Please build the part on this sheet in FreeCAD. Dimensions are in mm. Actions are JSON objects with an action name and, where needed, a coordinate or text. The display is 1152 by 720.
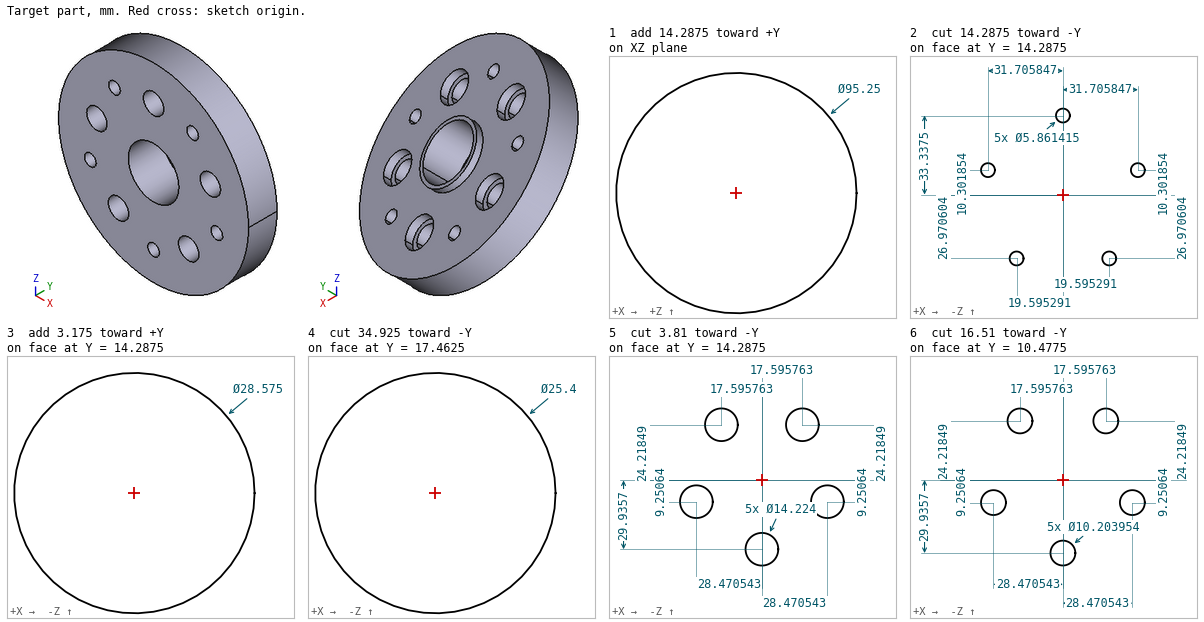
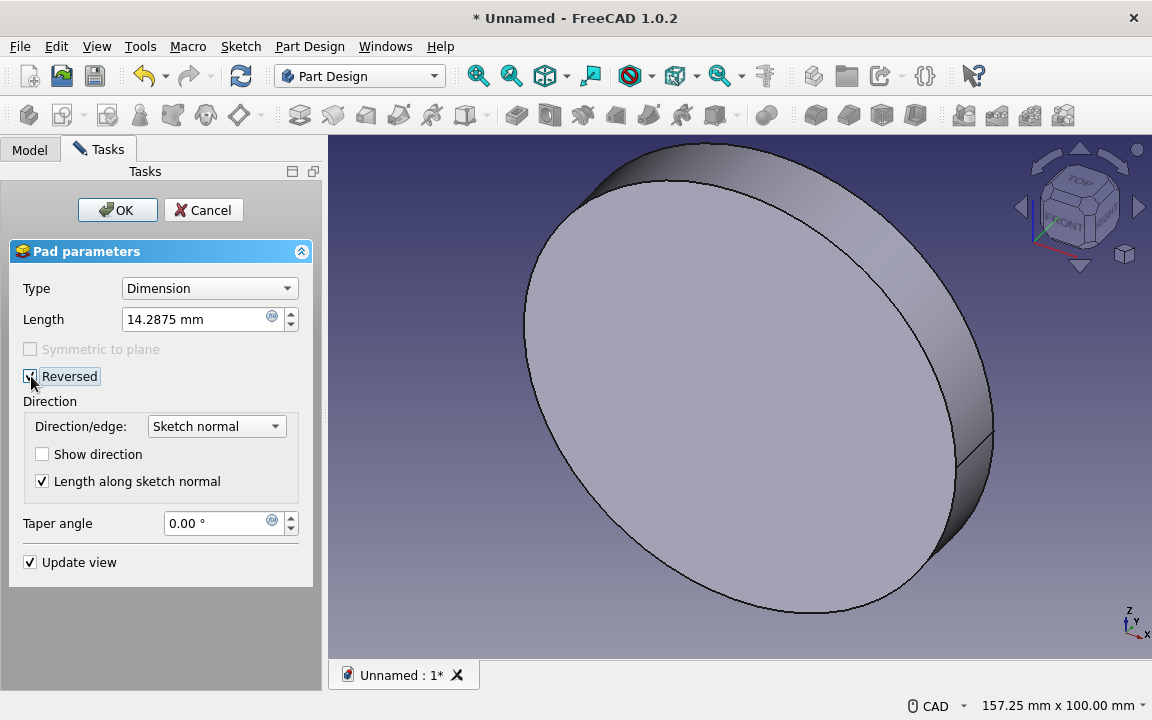
{"action": "left_click", "coordinate": [118, 210]}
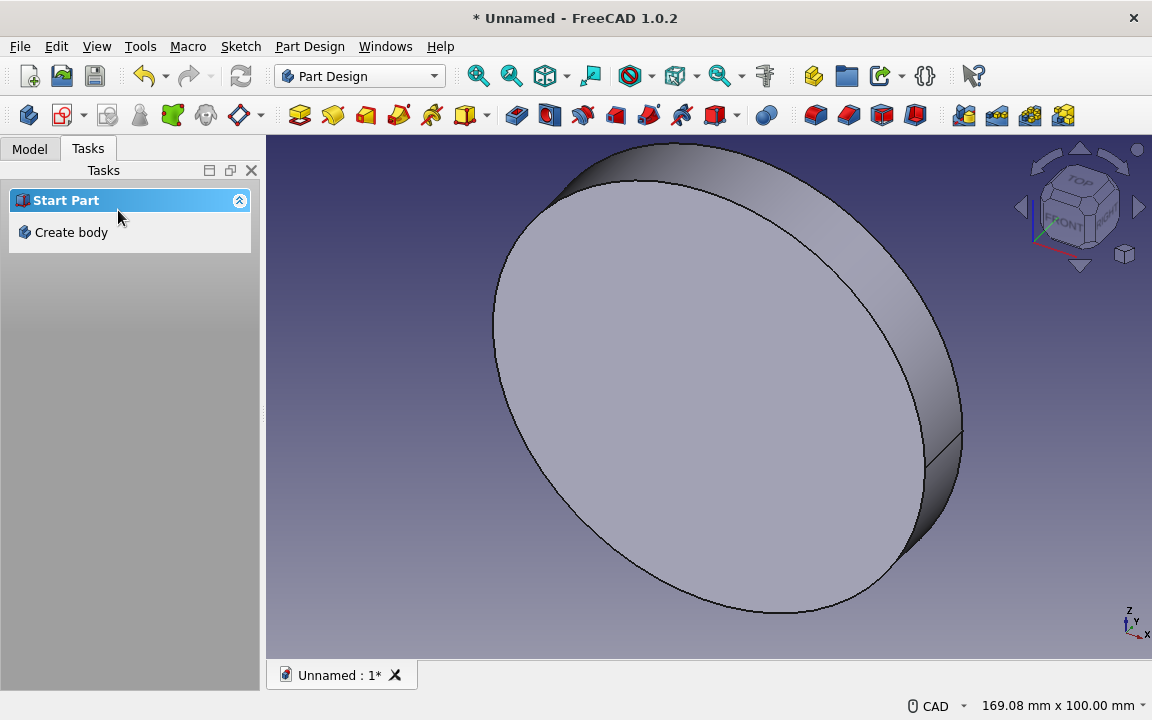
{"action": "left_click", "coordinate": [479, 76]}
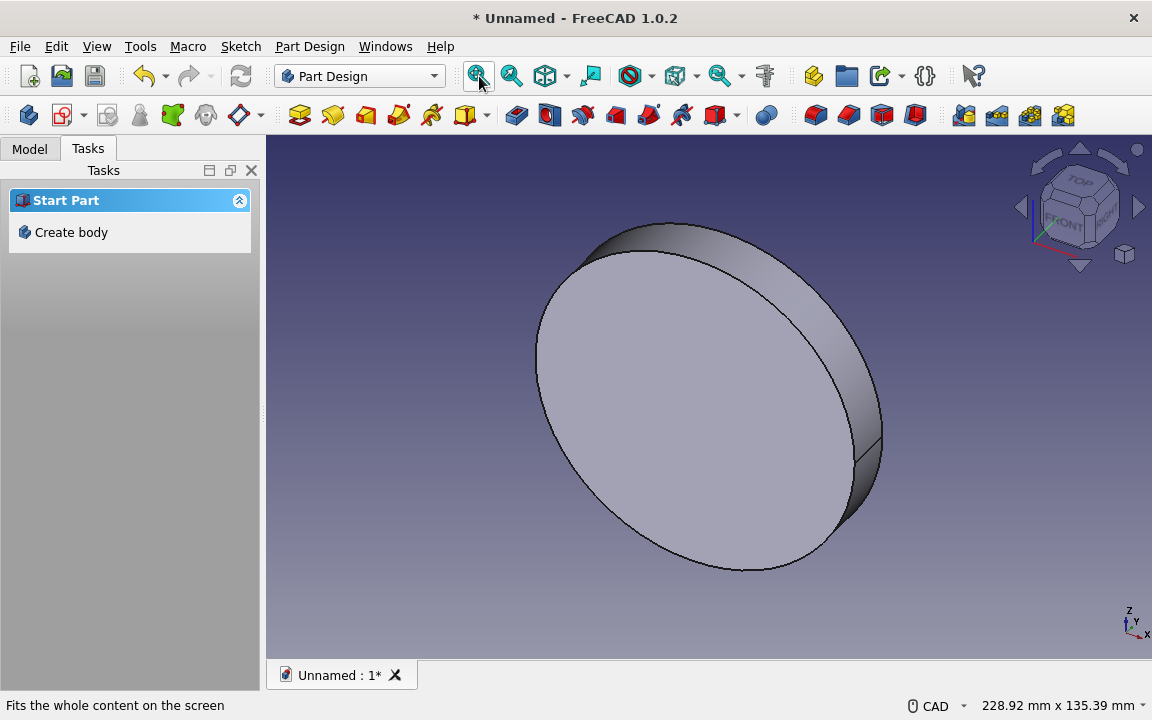
{"action": "key", "text": "4"}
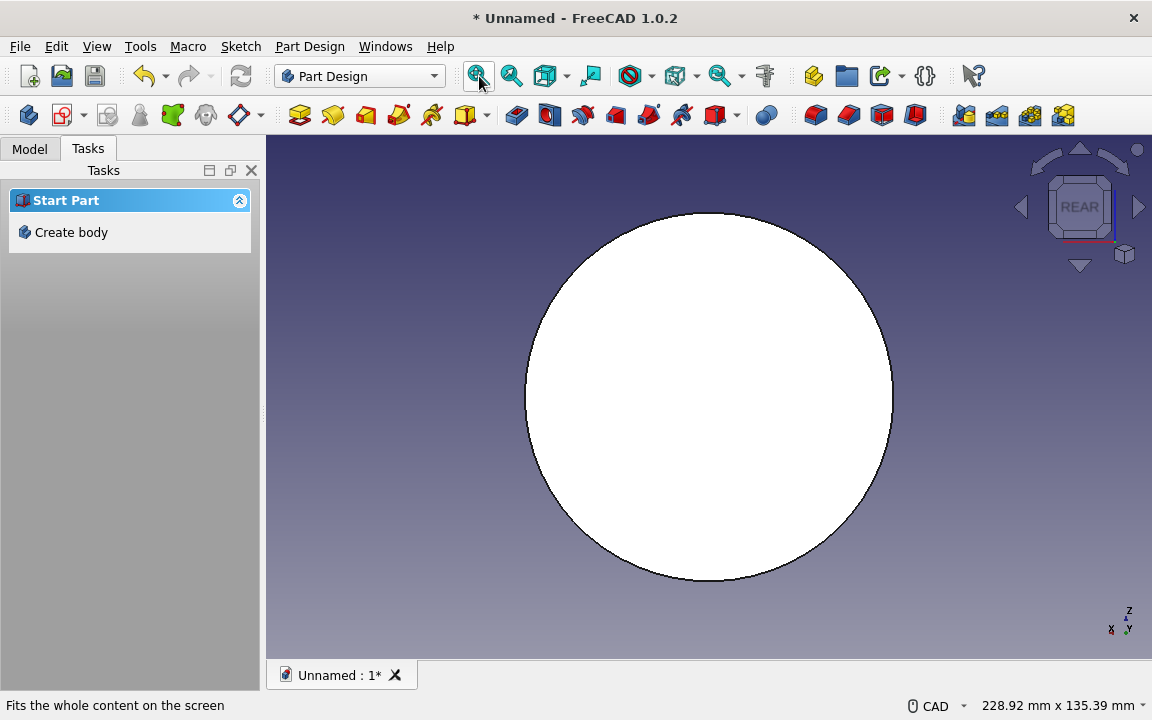
{"action": "left_click", "coordinate": [709, 396]}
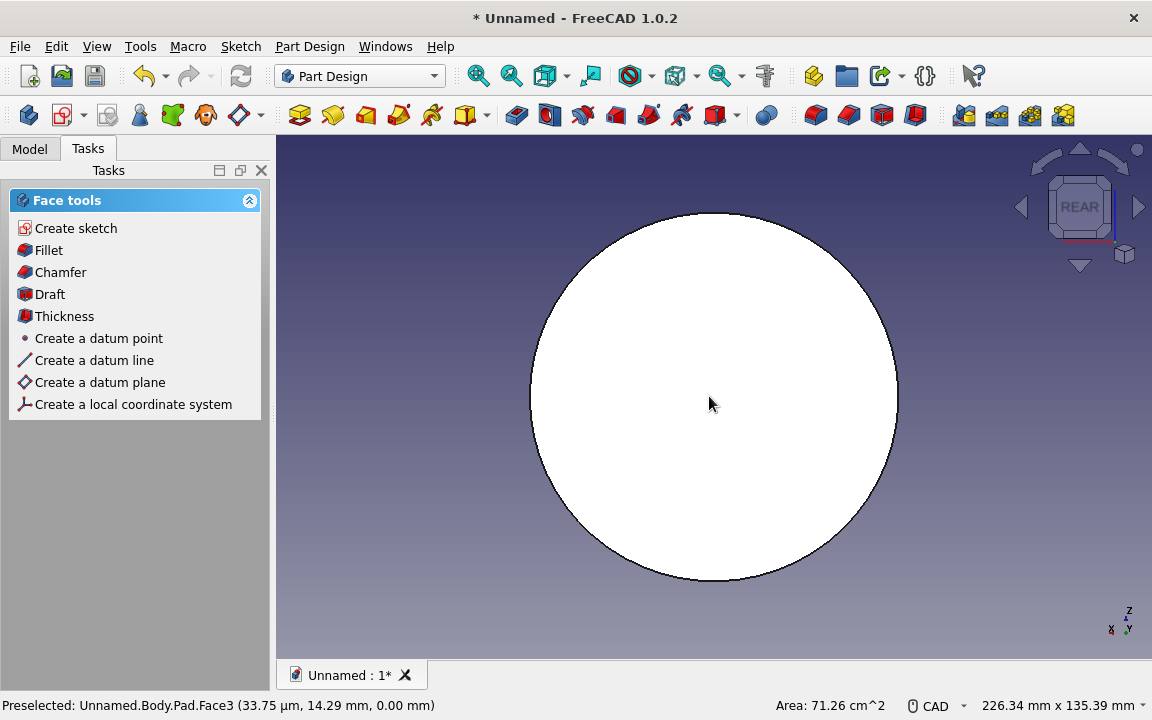
{"action": "left_click", "coordinate": [62, 116]}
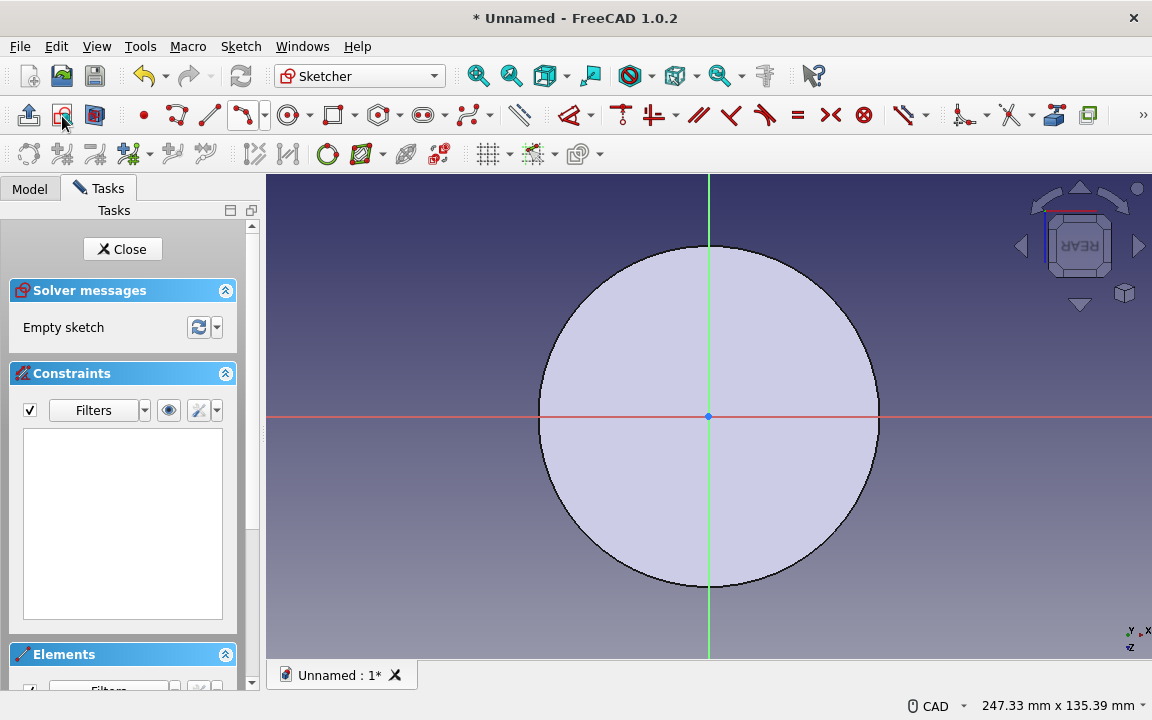
{"action": "left_click", "coordinate": [288, 116]}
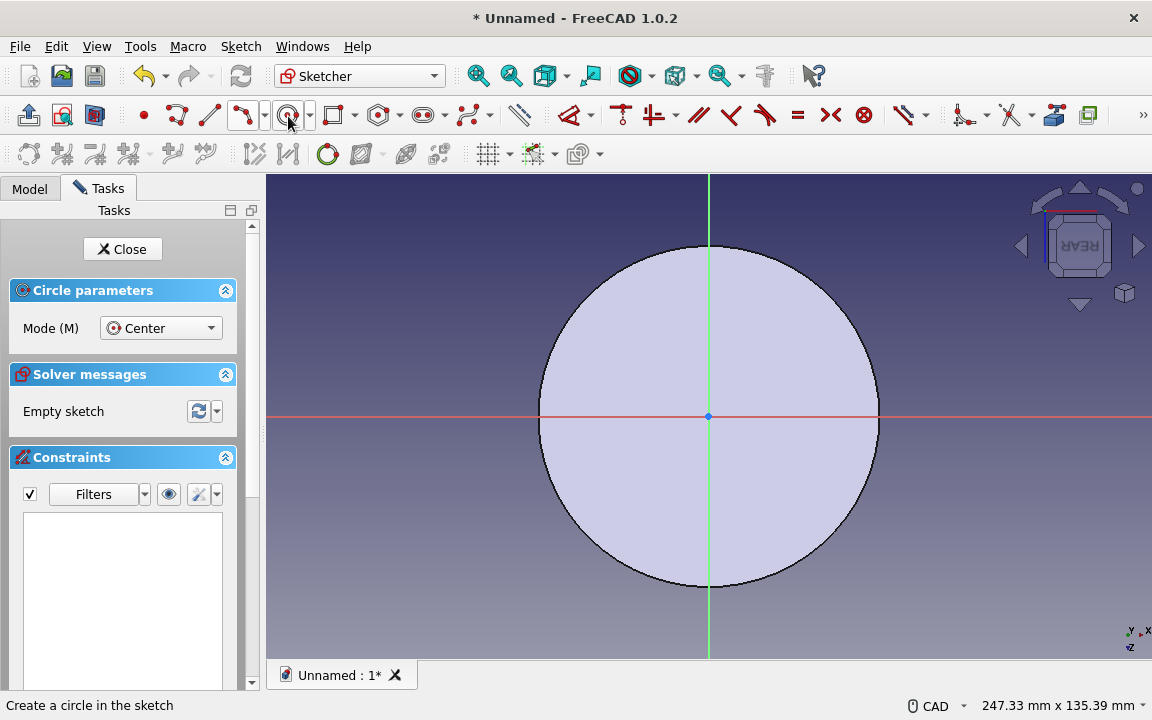
{"action": "scroll", "coordinate": [709, 297], "scroll_direction": "up", "scroll_amount": 4}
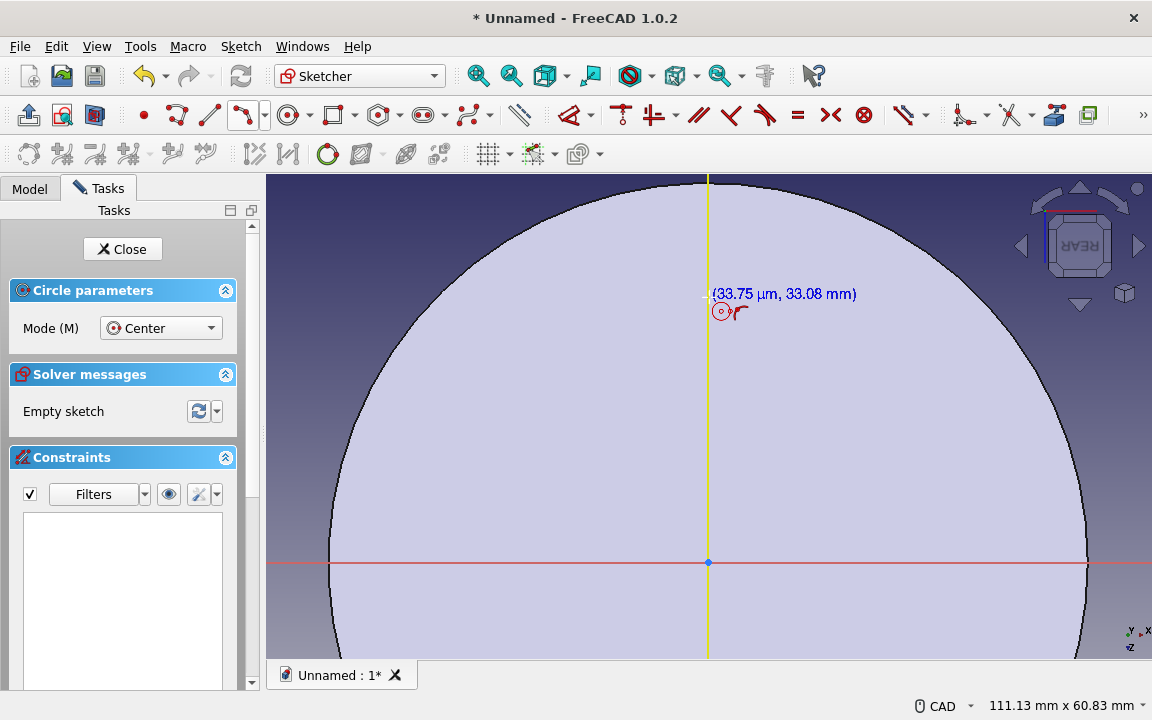
{"action": "left_click", "coordinate": [708, 297]}
{"action": "mouse_move", "coordinate": [725, 280]}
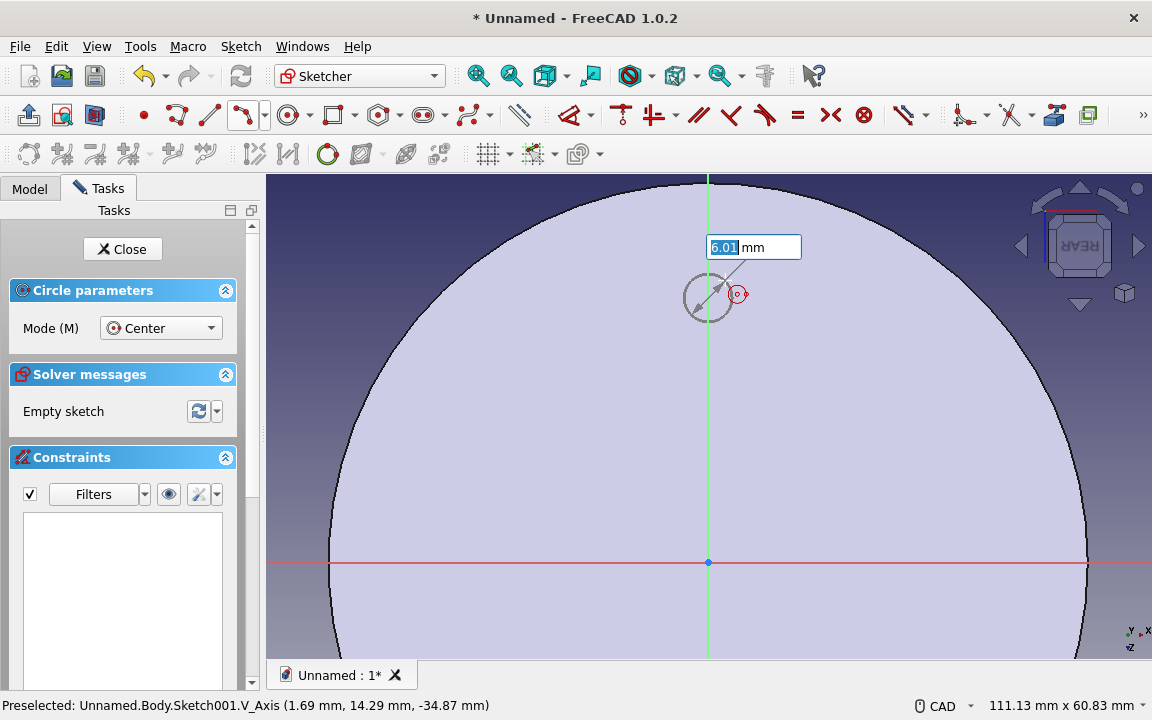
{"action": "type", "text": "5.861415"}
{"action": "key", "text": "Return"}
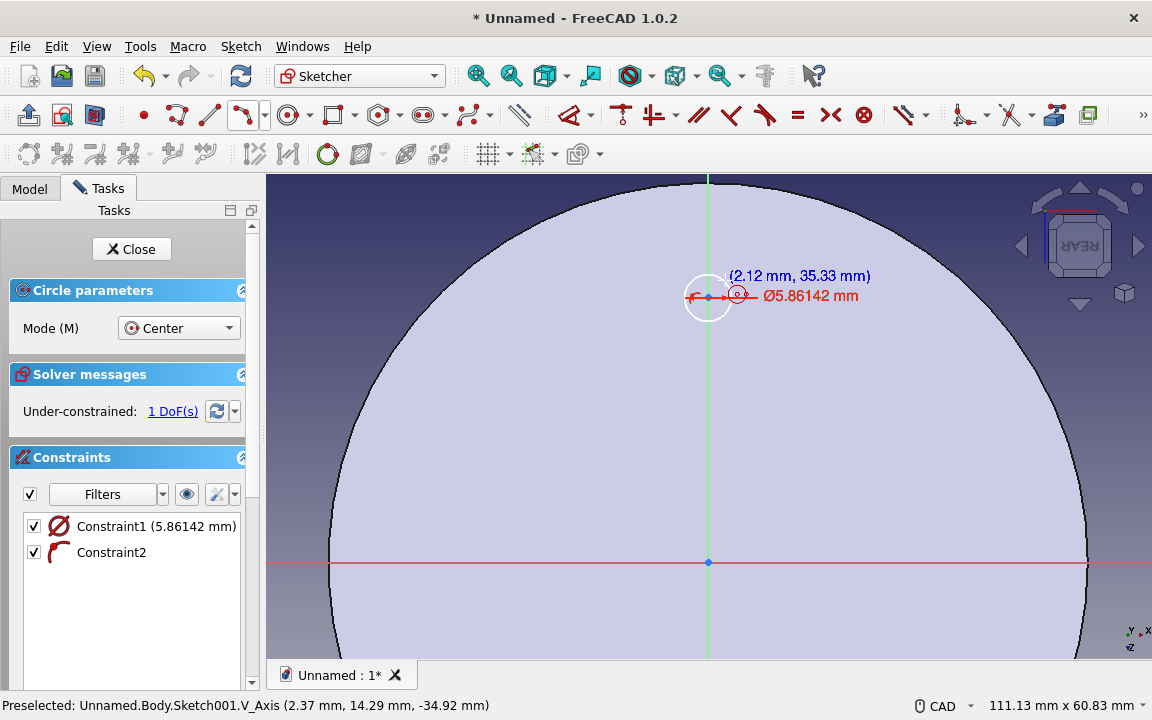
{"action": "left_click", "coordinate": [961, 481]}
{"action": "mouse_move", "coordinate": [977, 464]}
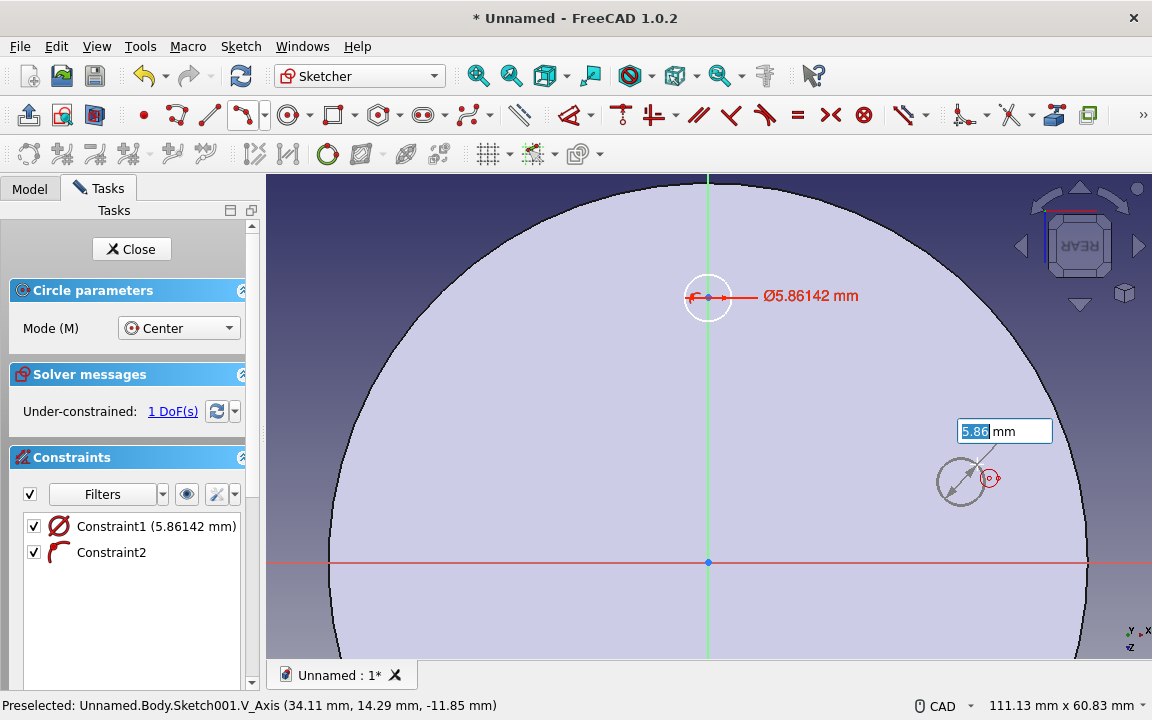
{"action": "type", "text": "5.861415"}
{"action": "key", "text": "Return"}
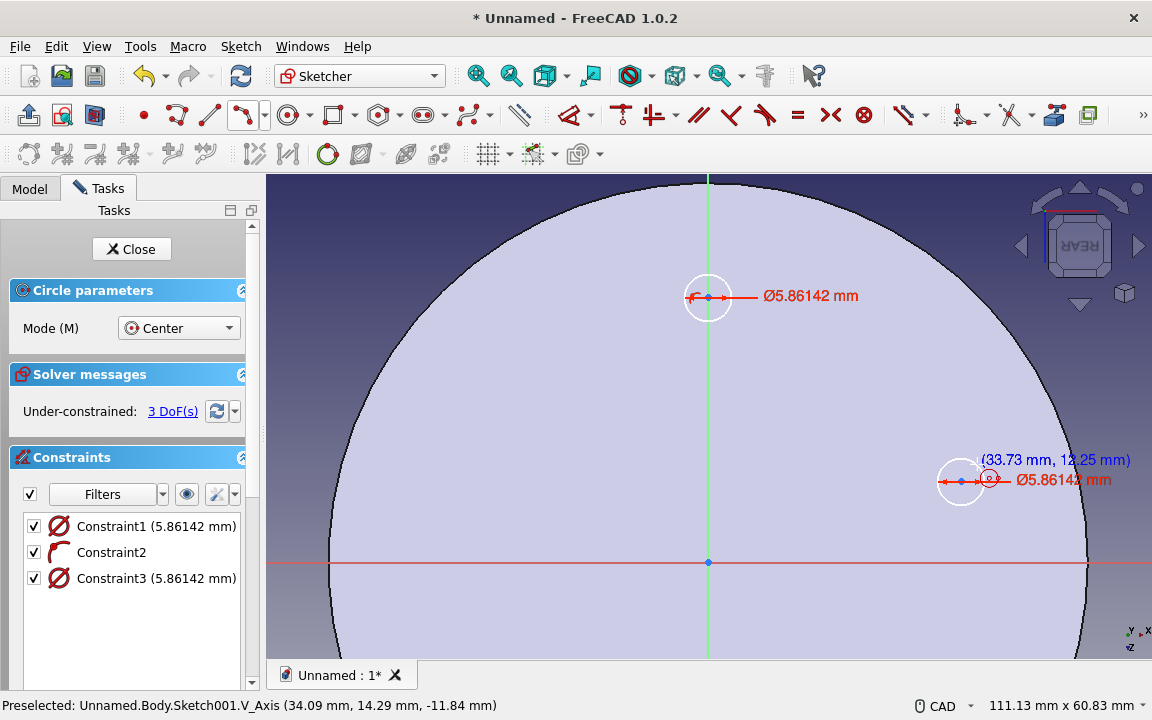
{"action": "scroll", "coordinate": [558, 270], "scroll_direction": "down", "scroll_amount": 3}